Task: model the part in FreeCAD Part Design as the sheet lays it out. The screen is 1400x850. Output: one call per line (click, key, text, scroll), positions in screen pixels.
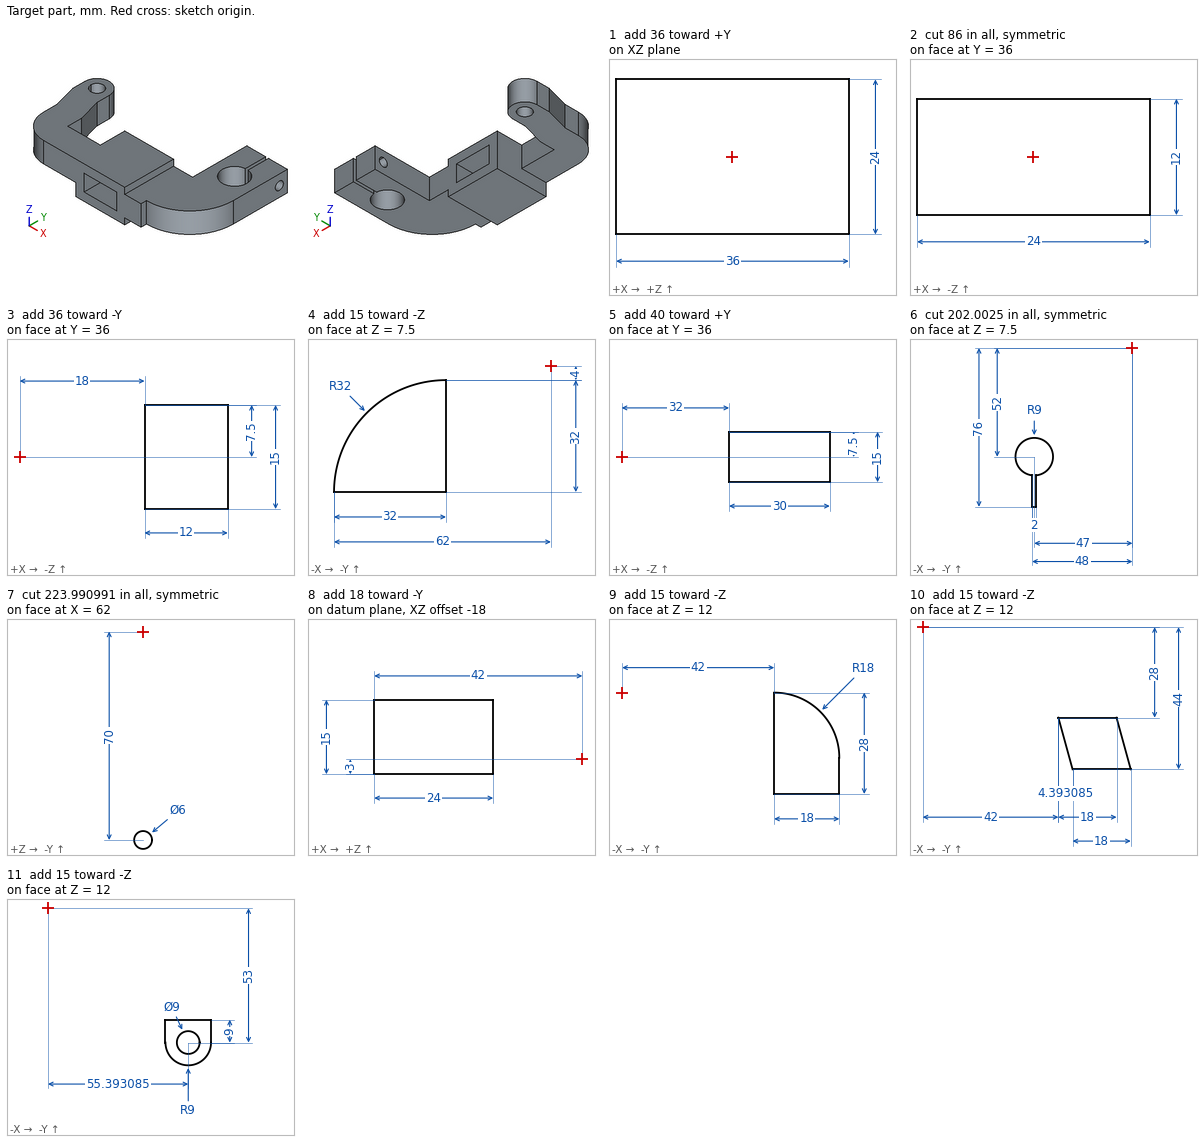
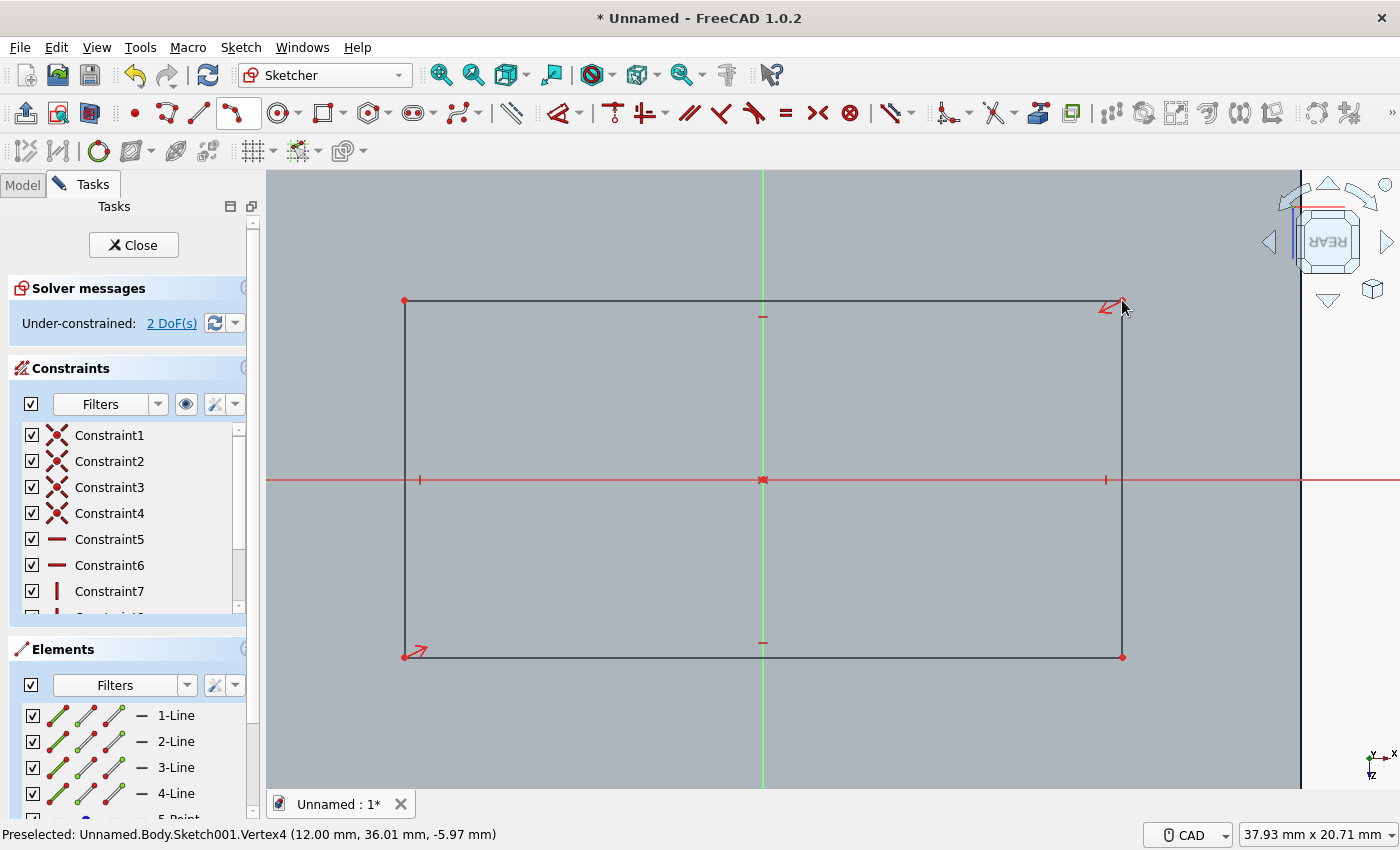
key(d)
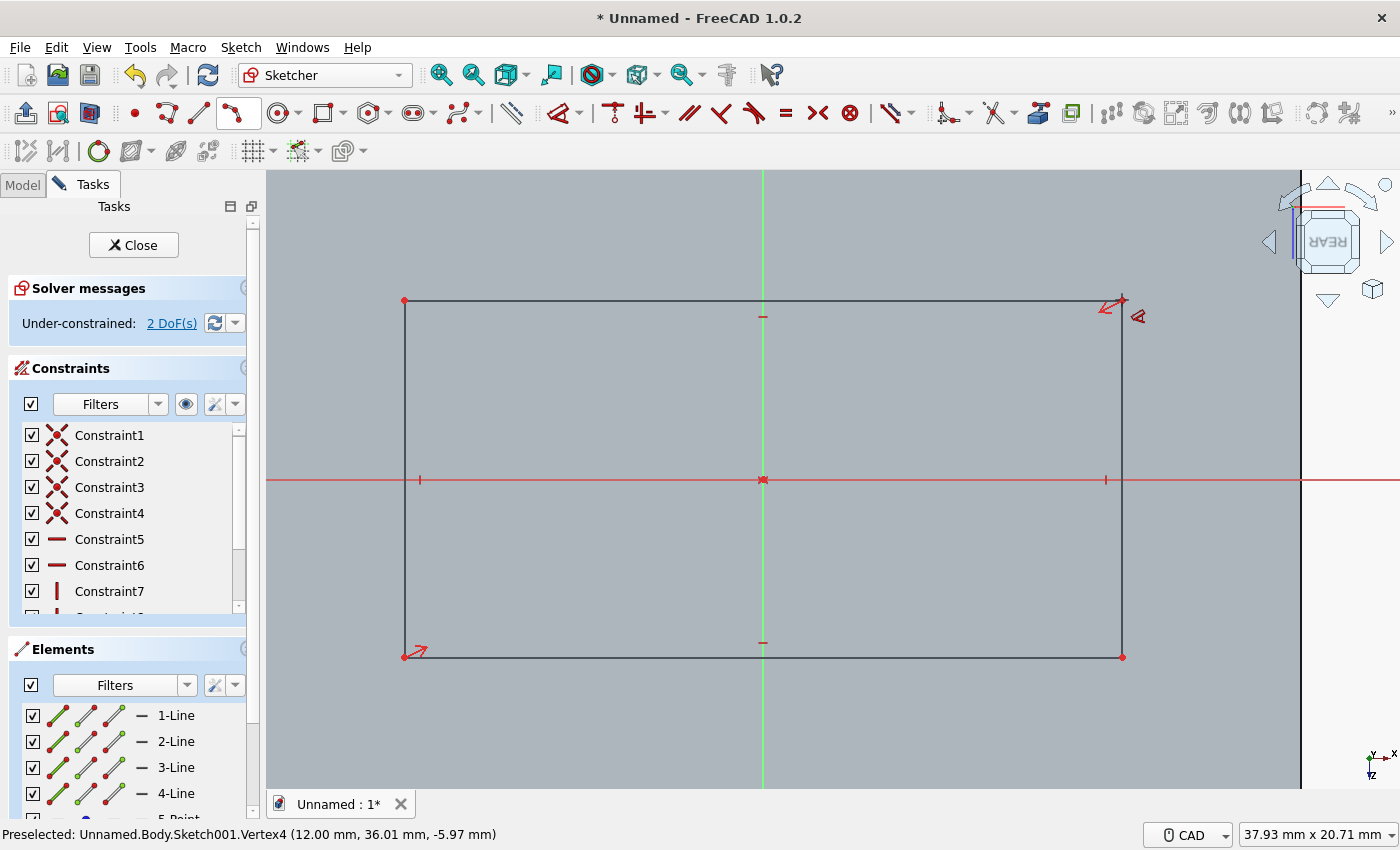
click(620, 658)
click(598, 692)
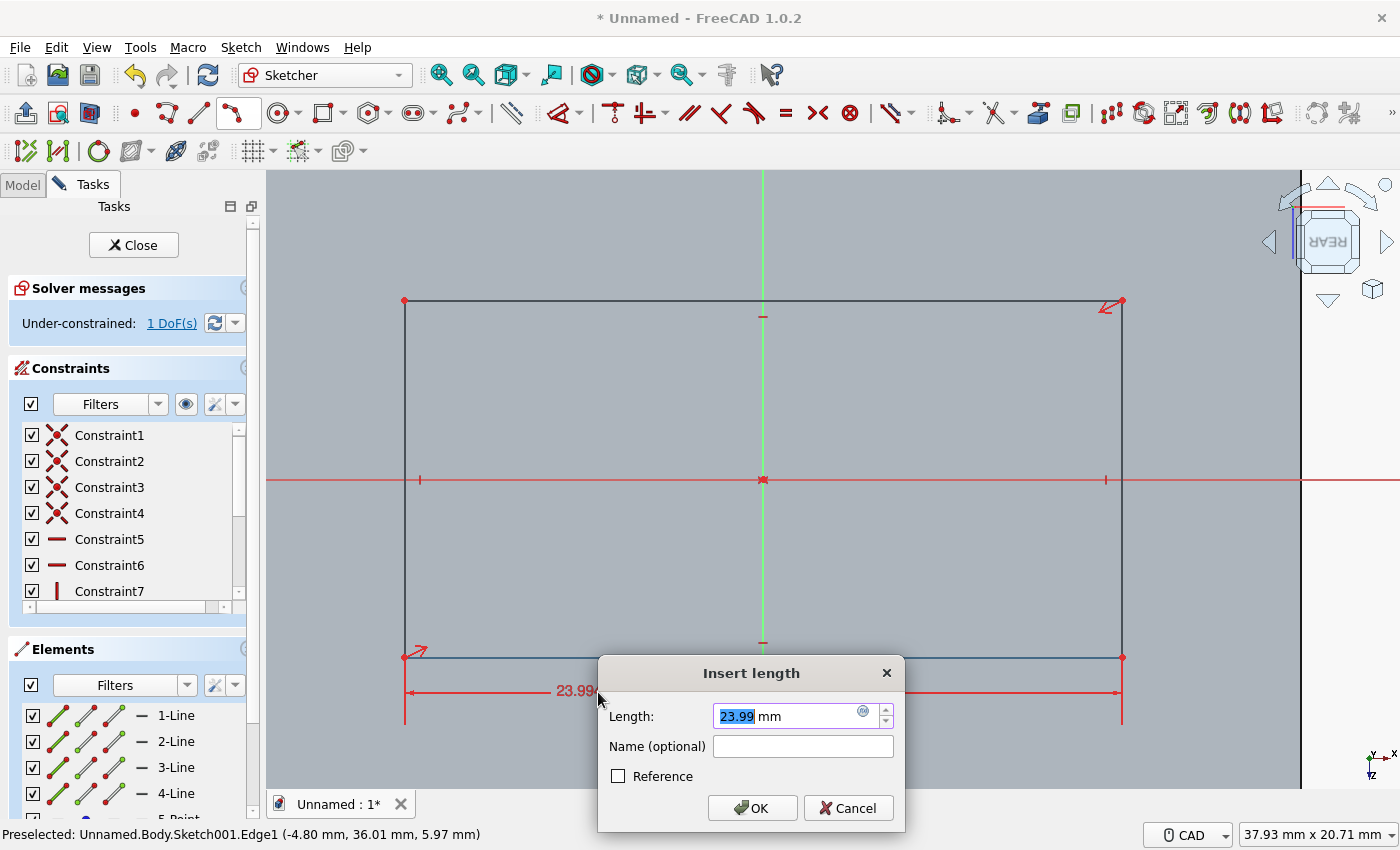
text(24)
key(Return)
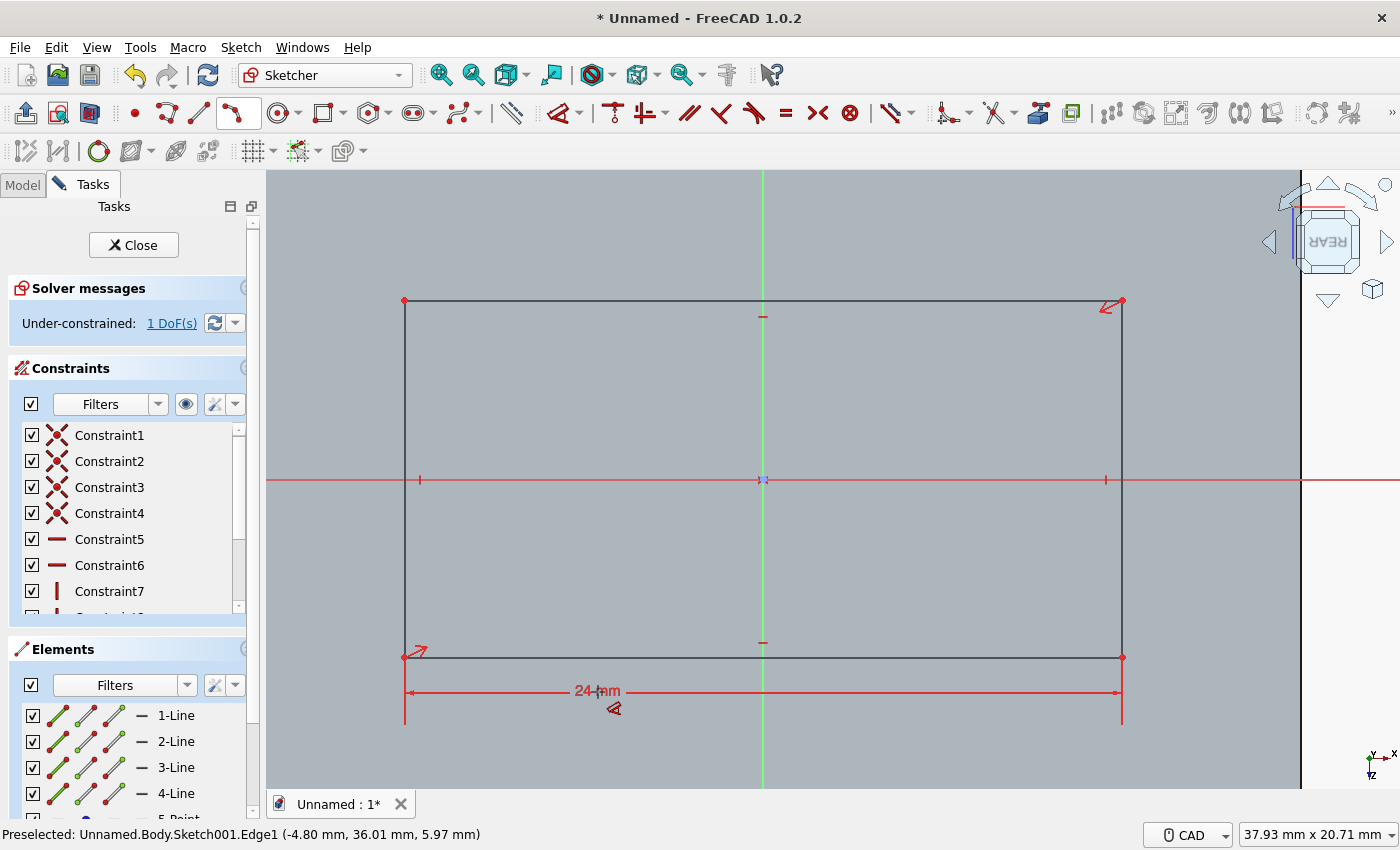
click(1122, 551)
click(1156, 397)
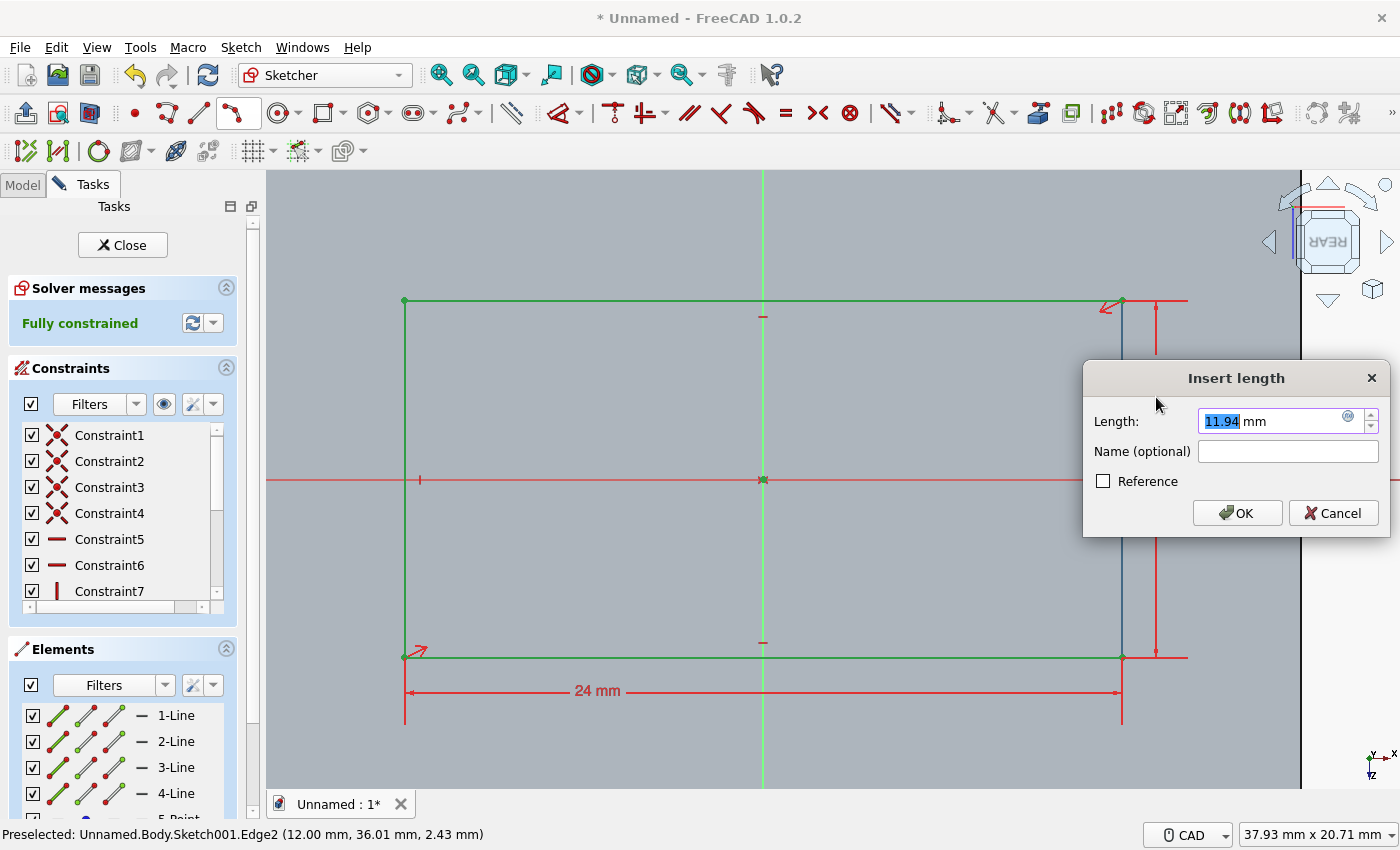
text(12)
key(Return)
key(Escape)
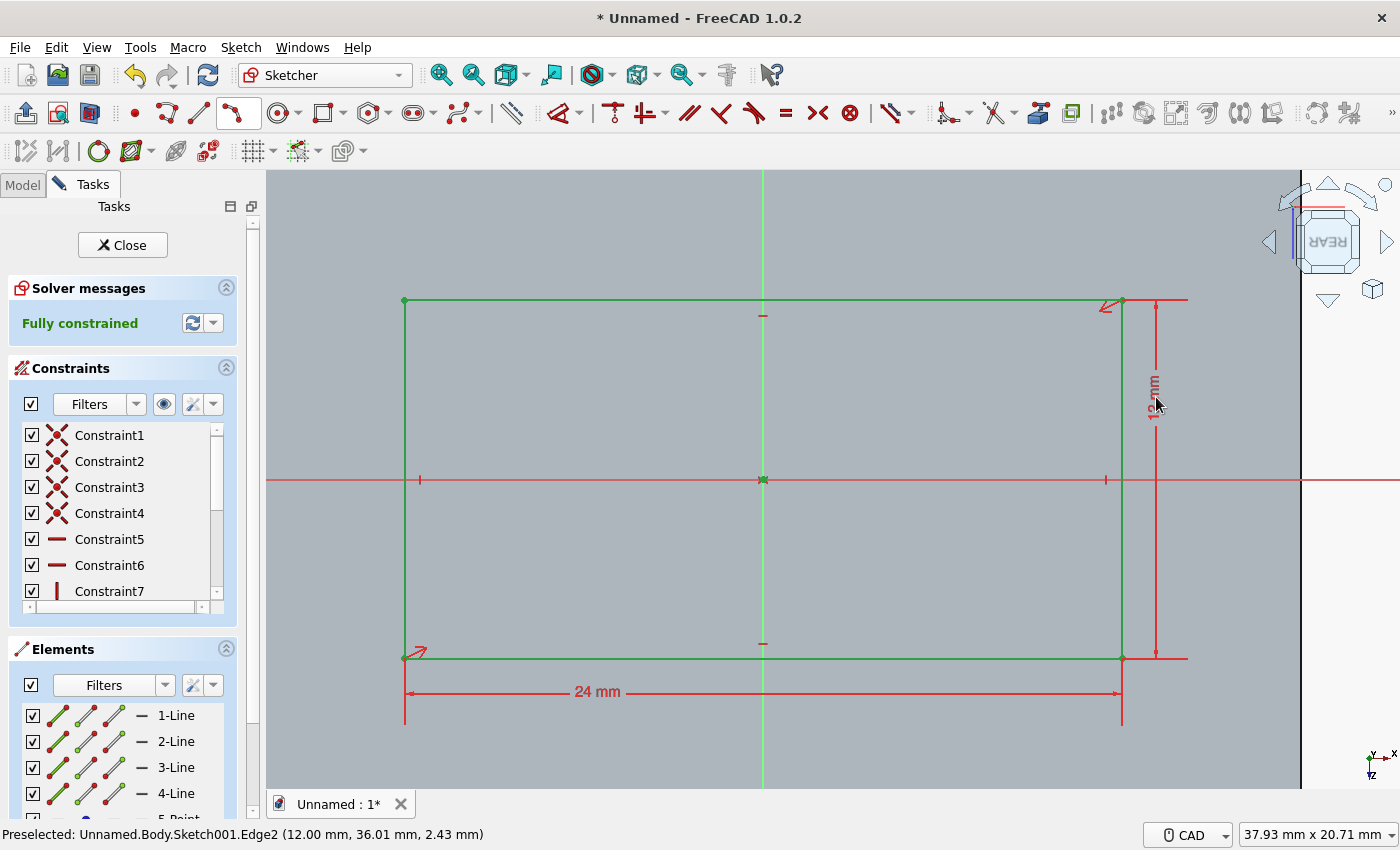
click(123, 245)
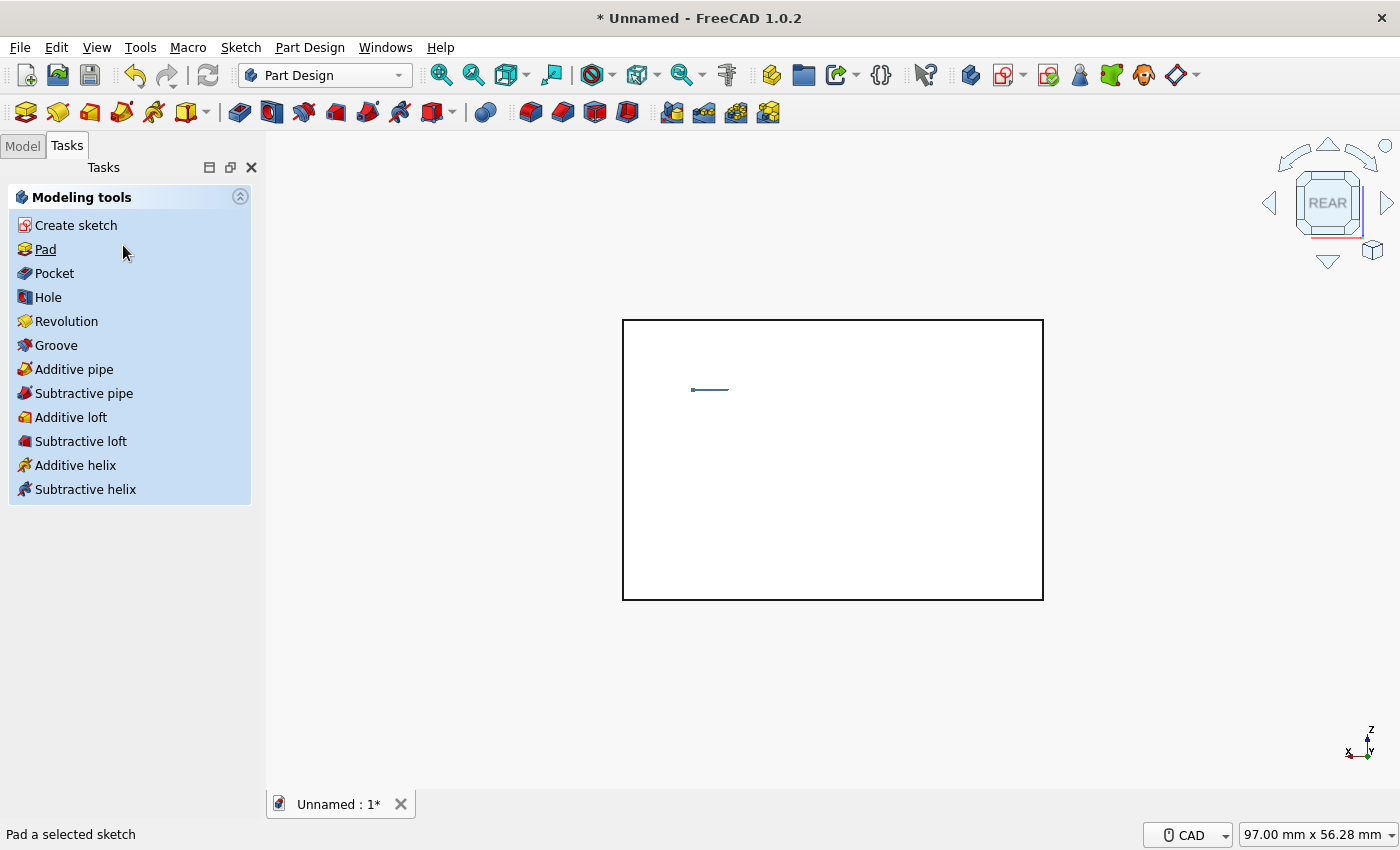
click(240, 112)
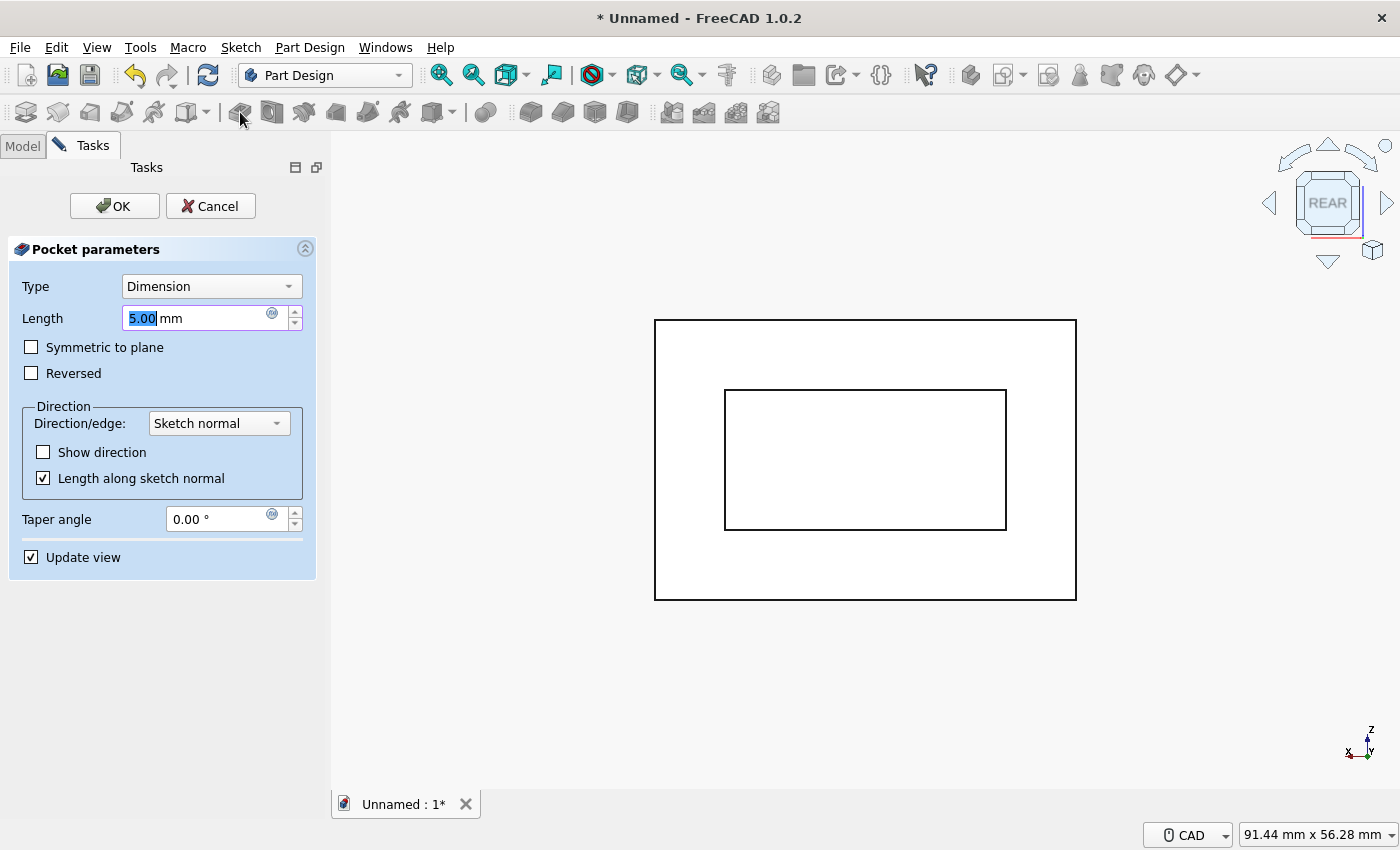
text(86)
key(Tab)